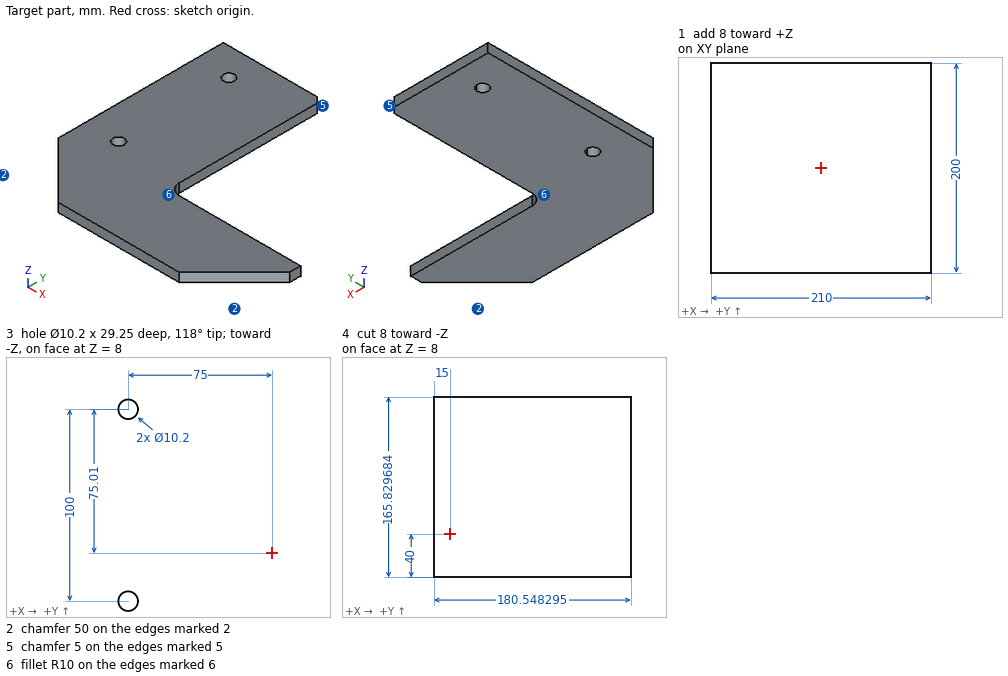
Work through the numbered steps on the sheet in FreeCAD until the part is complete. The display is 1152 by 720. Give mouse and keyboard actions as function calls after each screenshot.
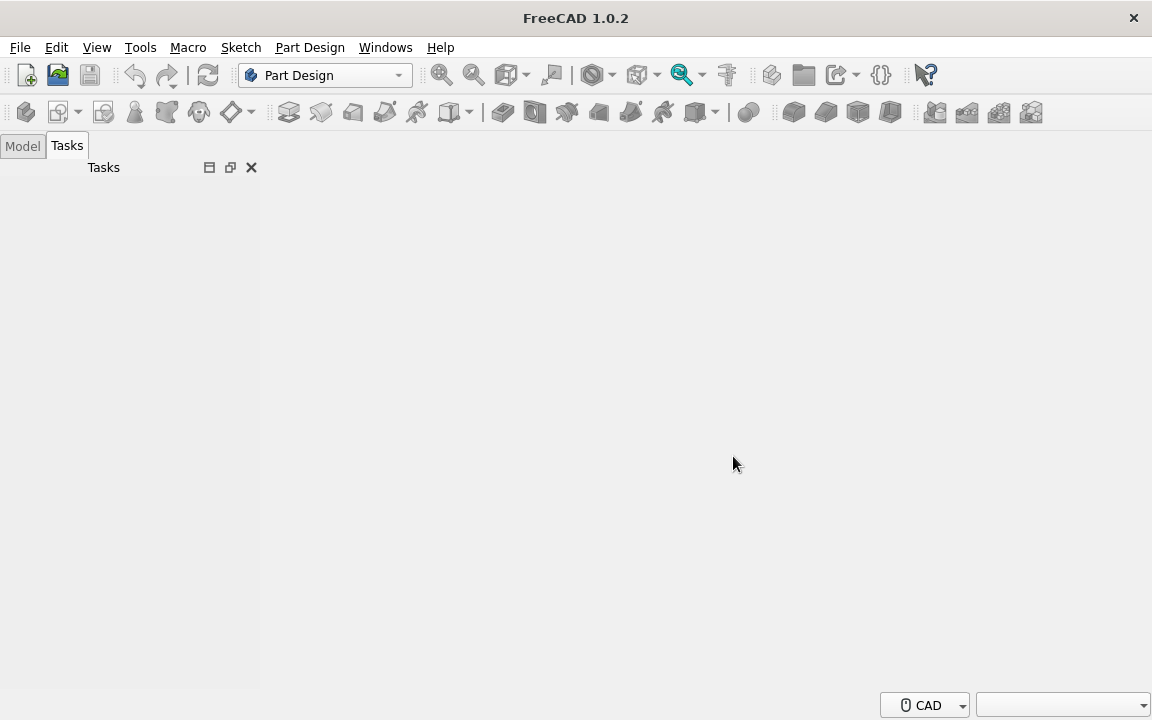
click(26, 76)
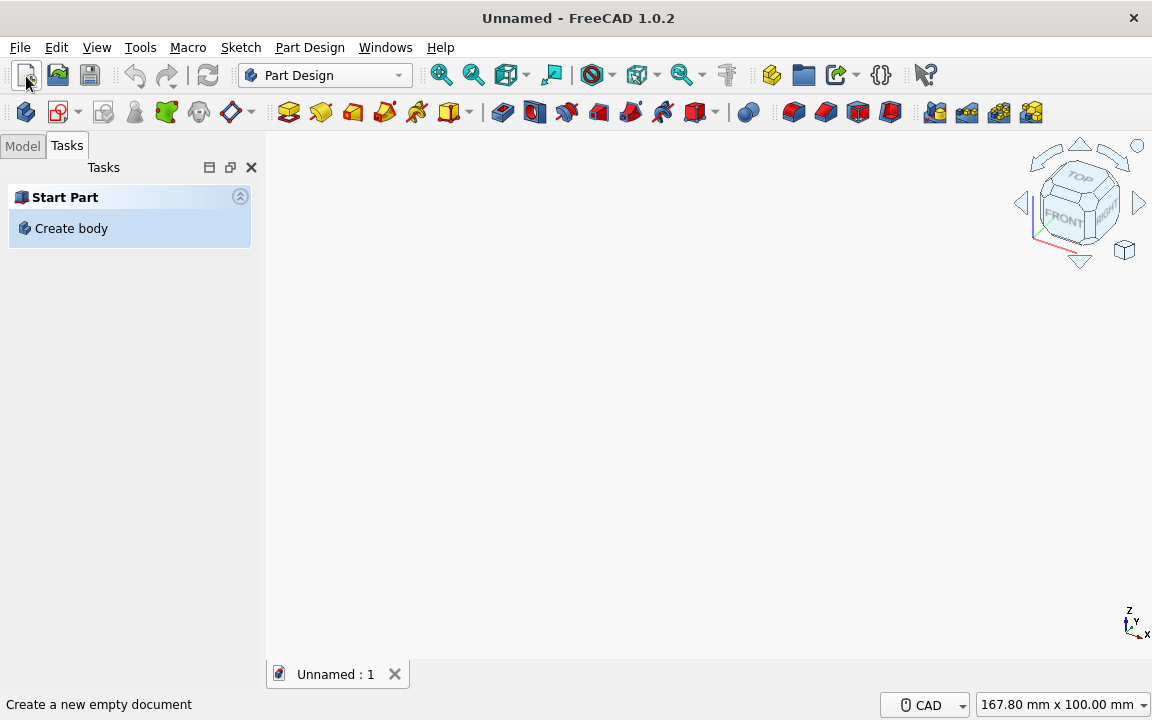
click(58, 112)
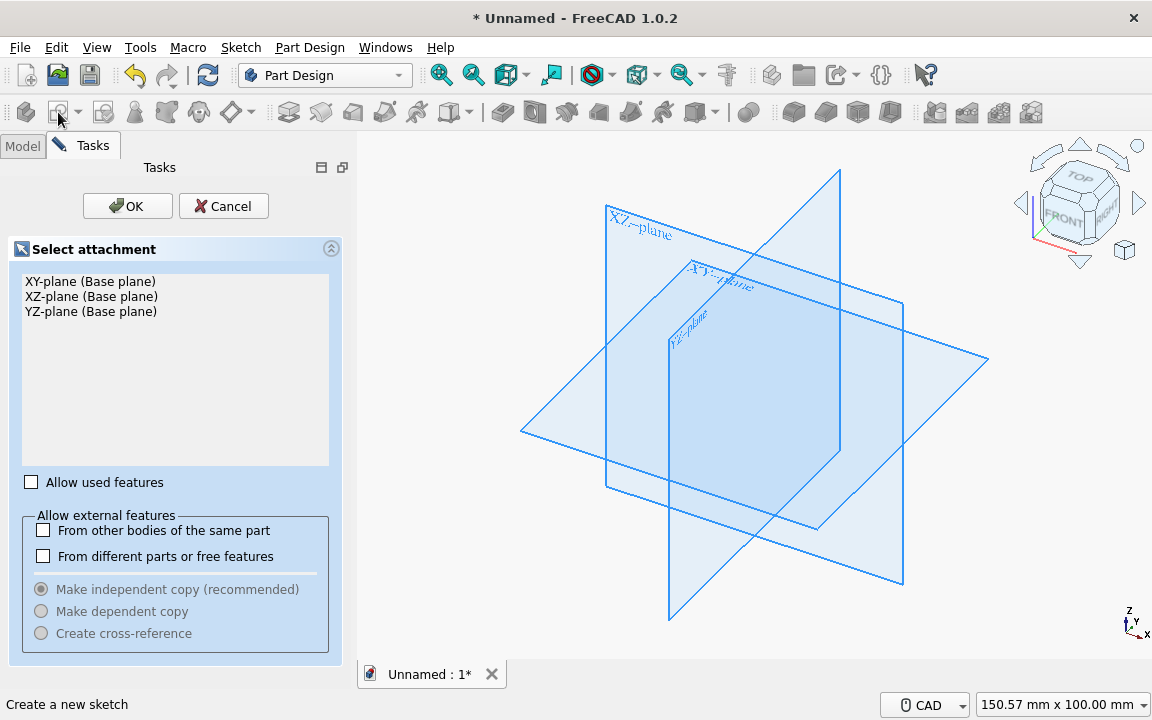
click(82, 282)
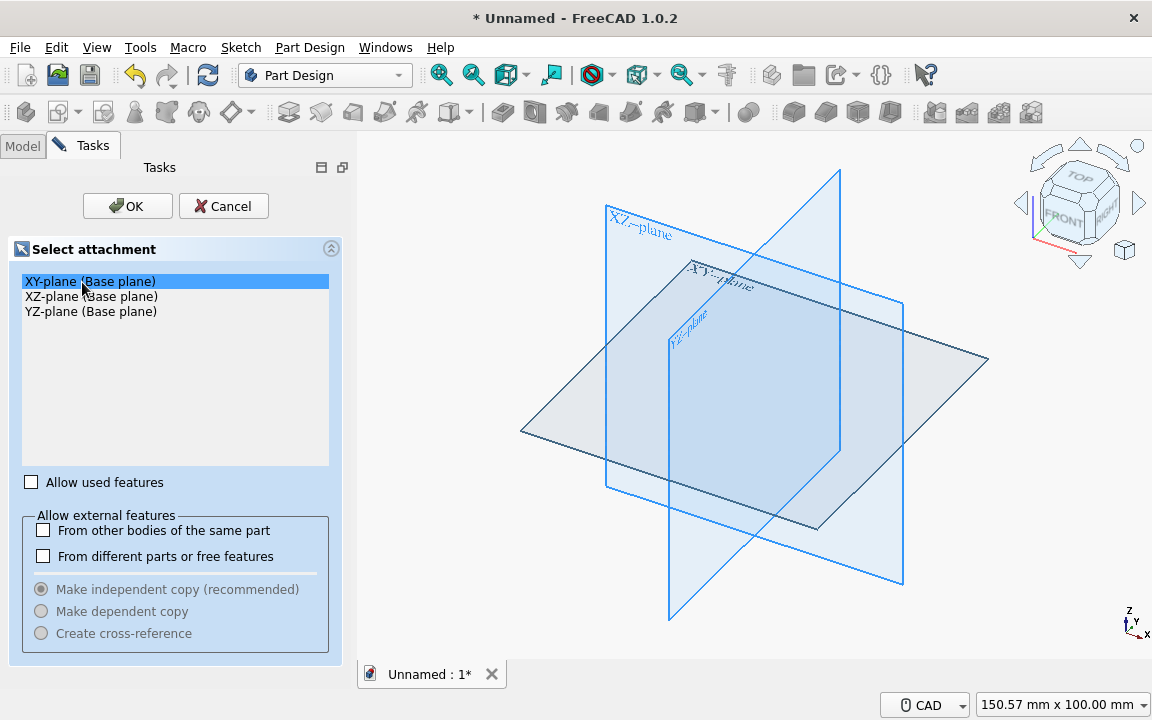
click(128, 206)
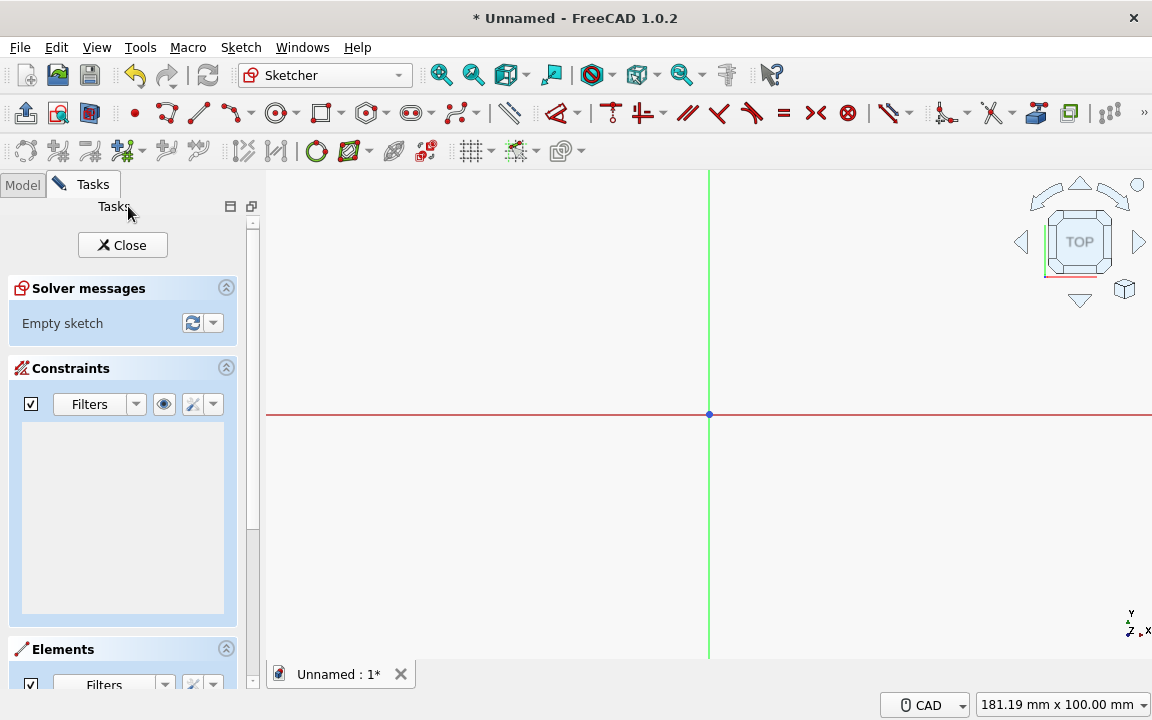
scroll(611, 414, down, 6)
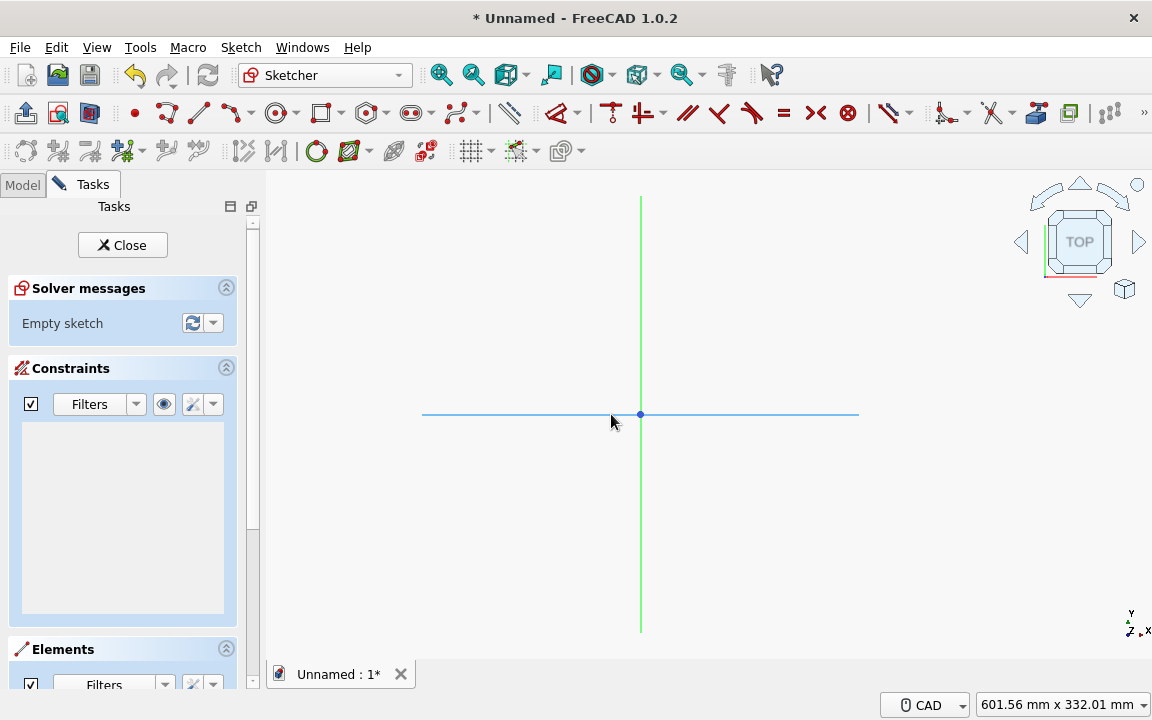
click(344, 114)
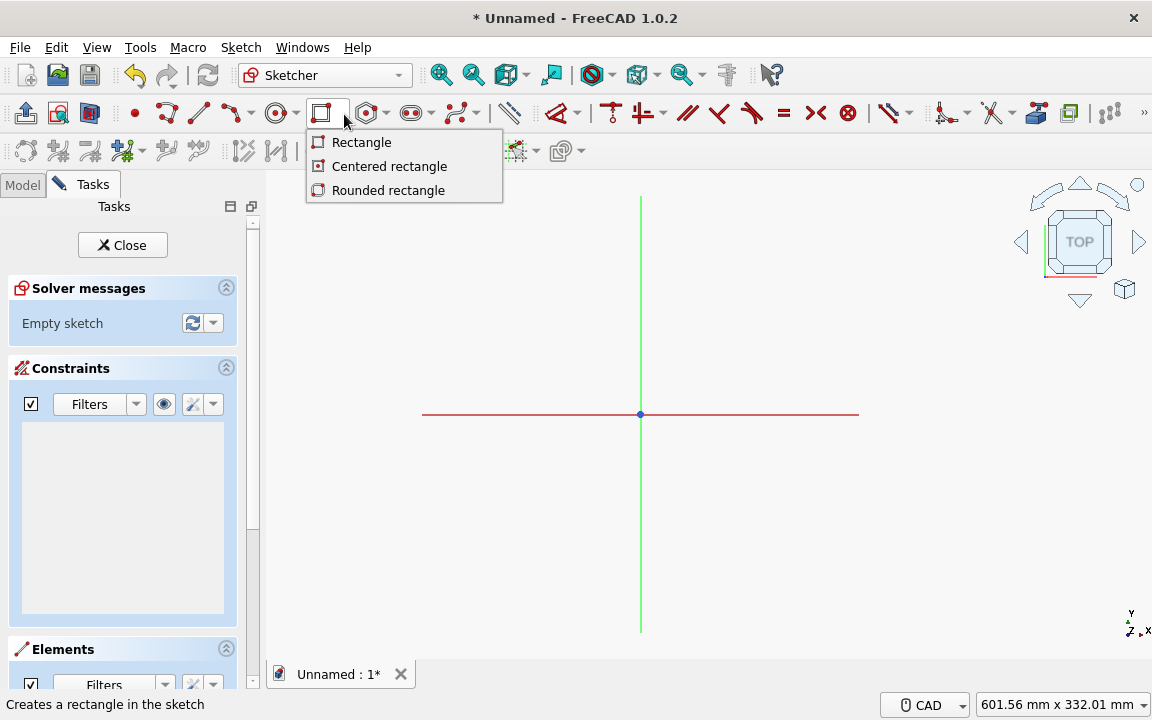
click(404, 166)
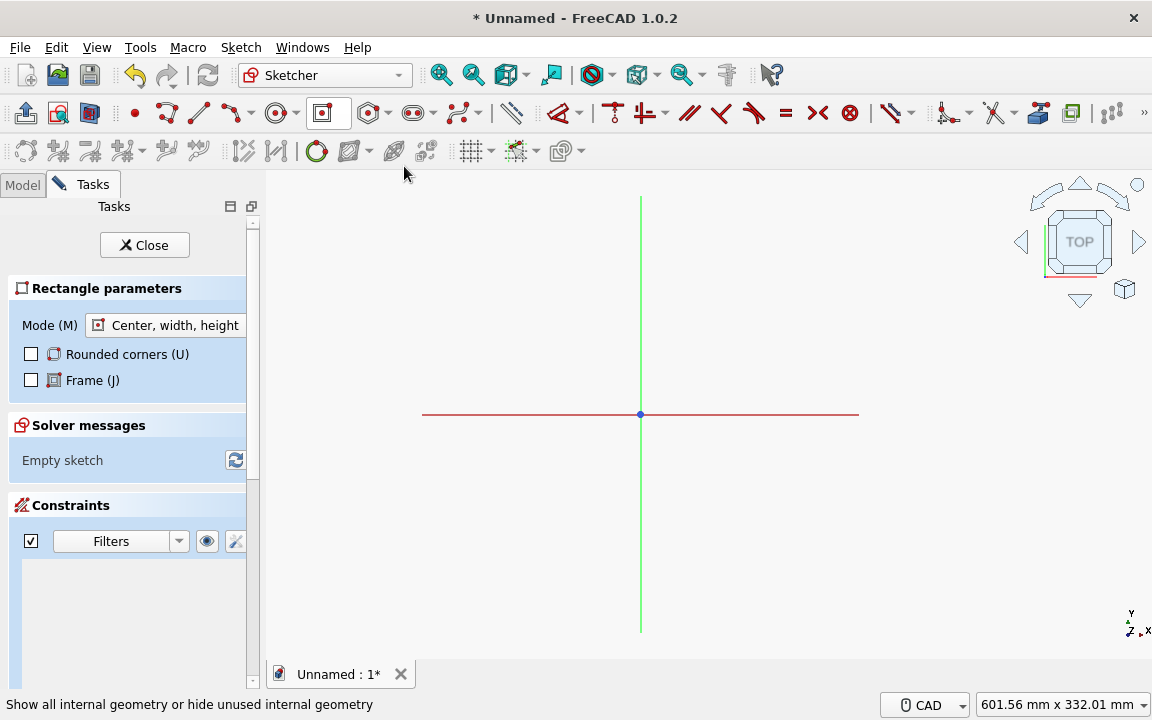
click(641, 414)
click(795, 267)
key(Escape)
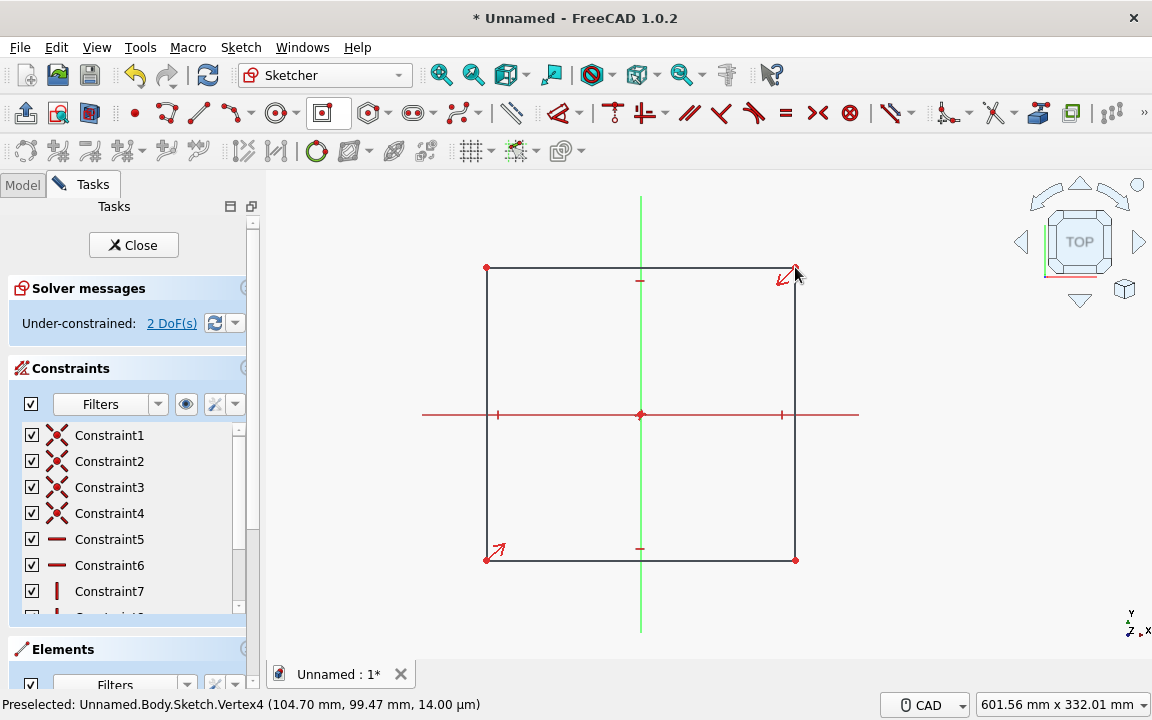
click(579, 561)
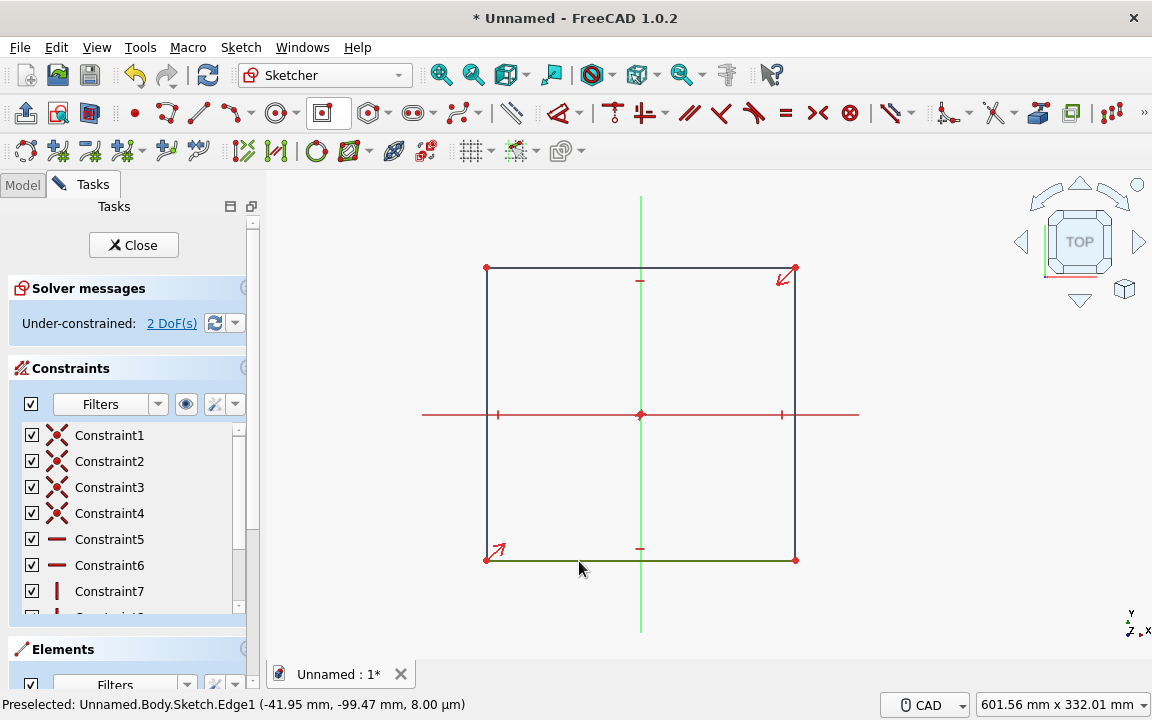
key(l)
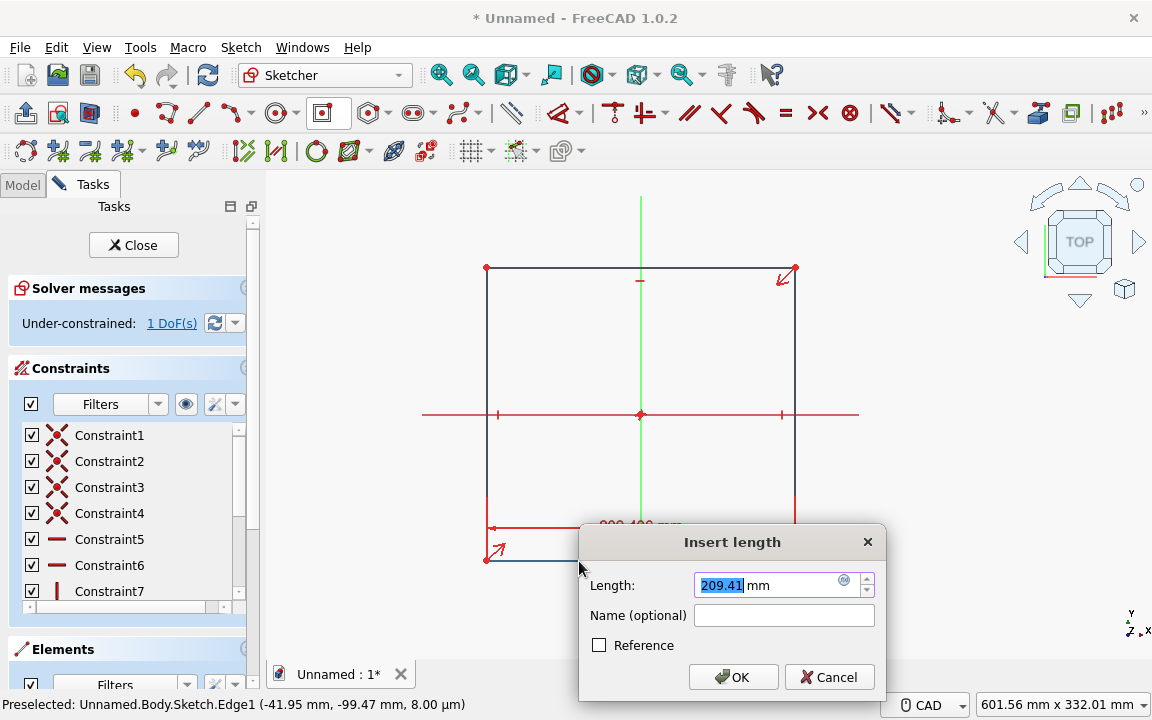
text(210)
key(Return)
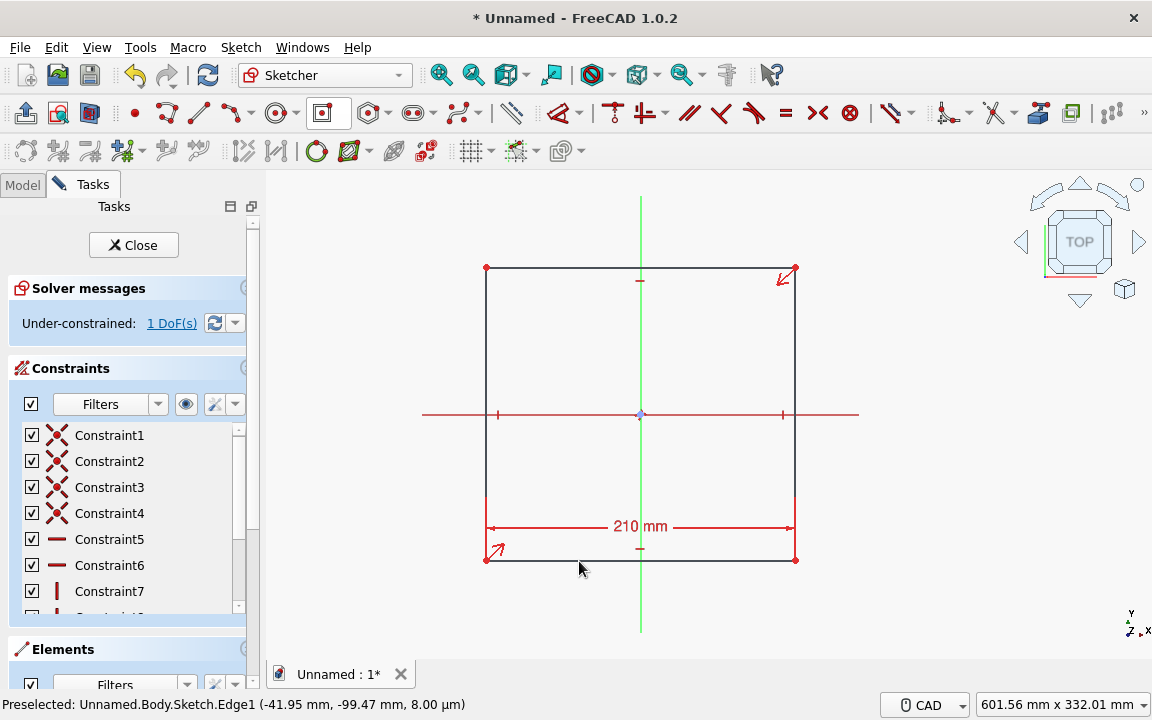
click(795, 473)